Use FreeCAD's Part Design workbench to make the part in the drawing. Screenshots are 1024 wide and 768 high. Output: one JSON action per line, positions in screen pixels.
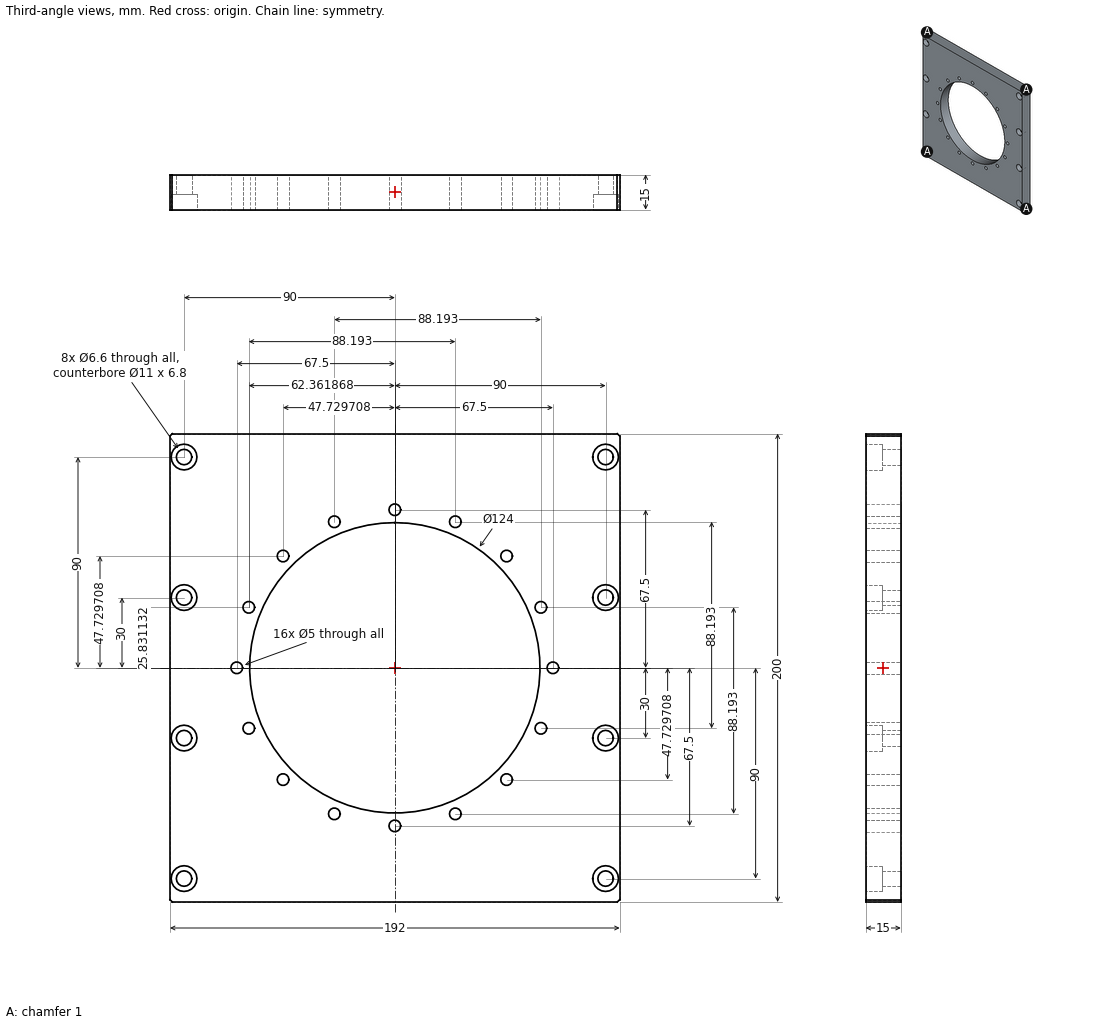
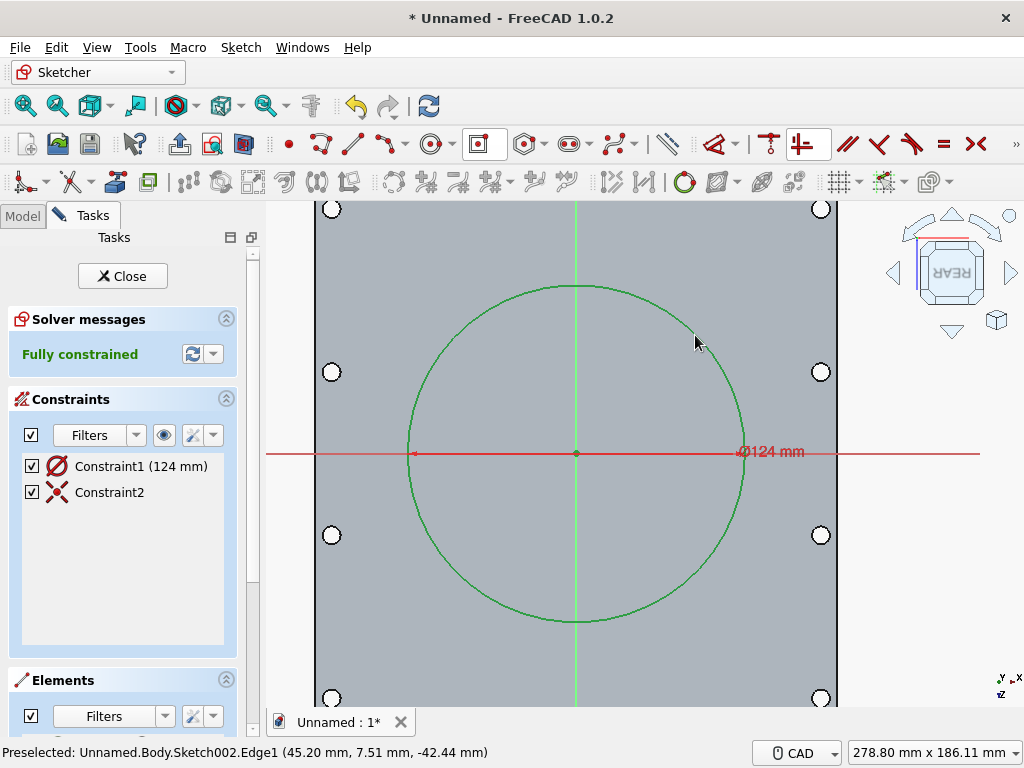
{"action": "left_click", "coordinate": [123, 276]}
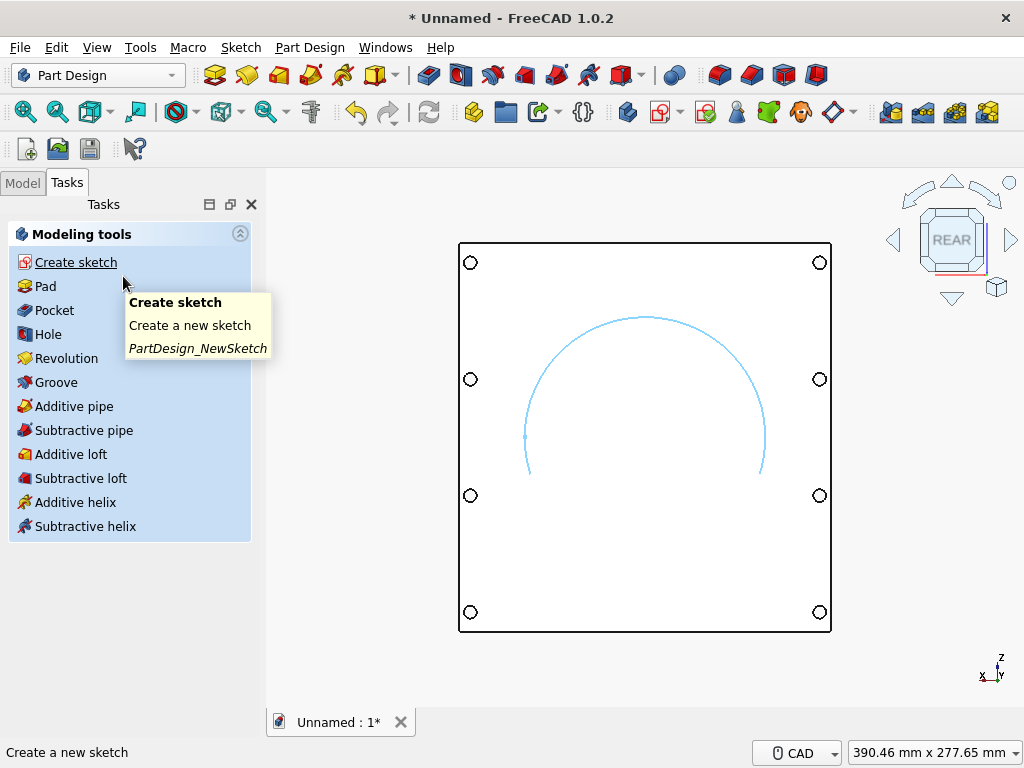
{"action": "left_click", "coordinate": [430, 76]}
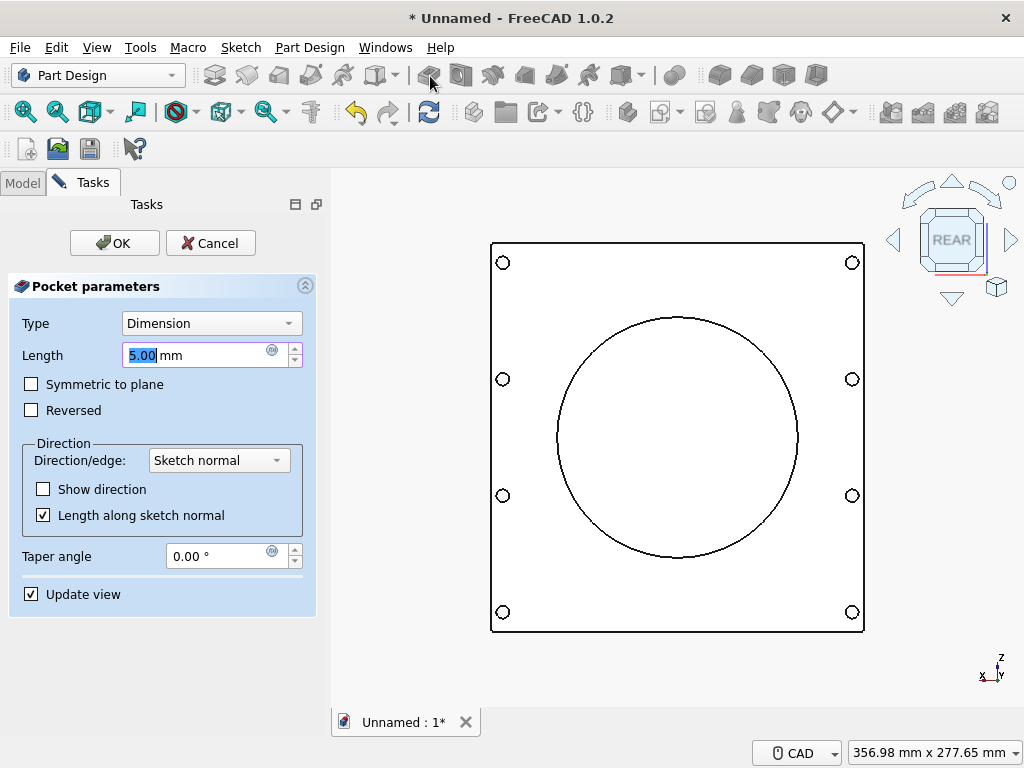
{"action": "type", "text": "15"}
{"action": "key", "text": "Tab"}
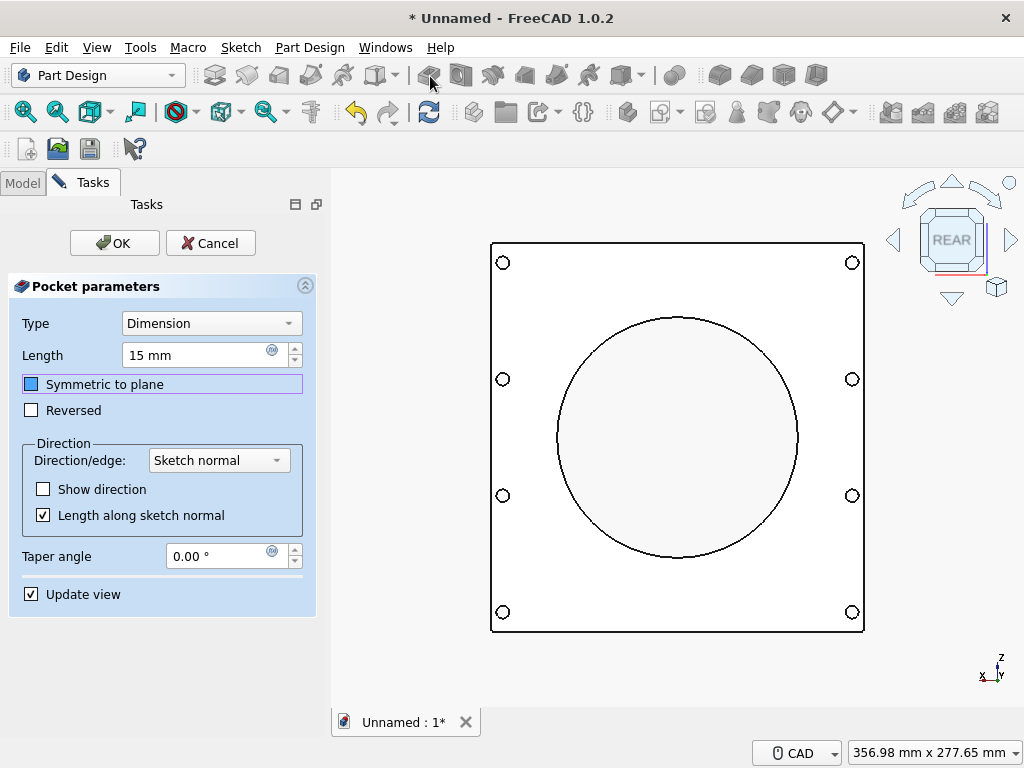
{"action": "left_click", "coordinate": [115, 243]}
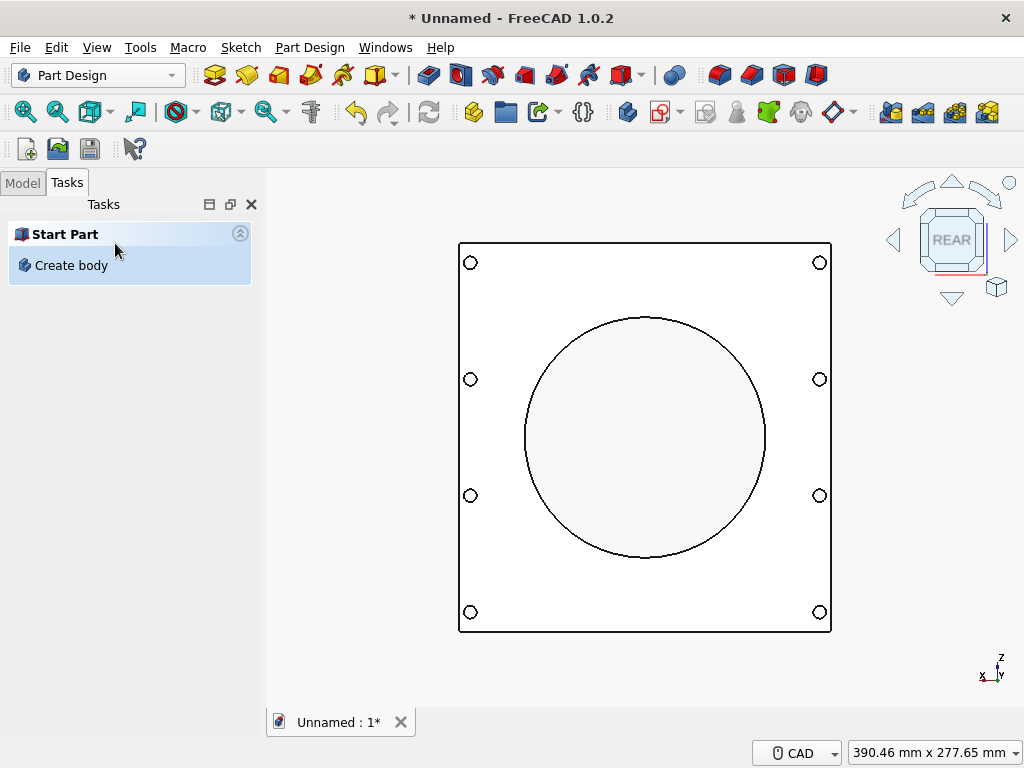
{"action": "key", "text": "0"}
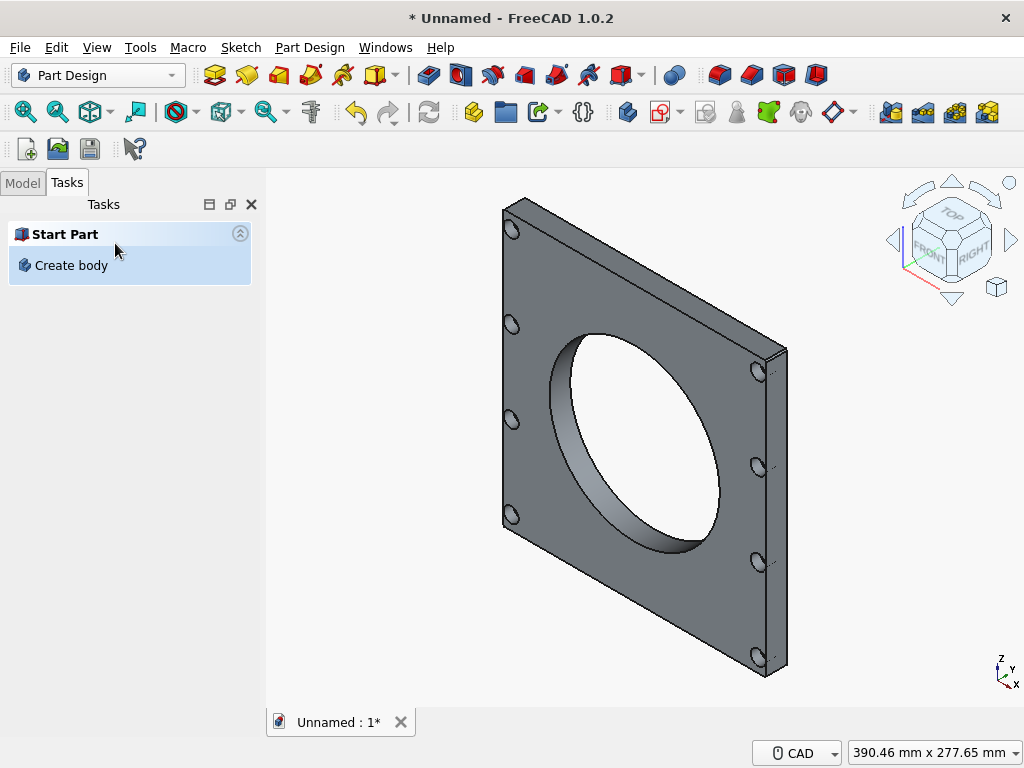
{"action": "left_click", "coordinate": [710, 395]}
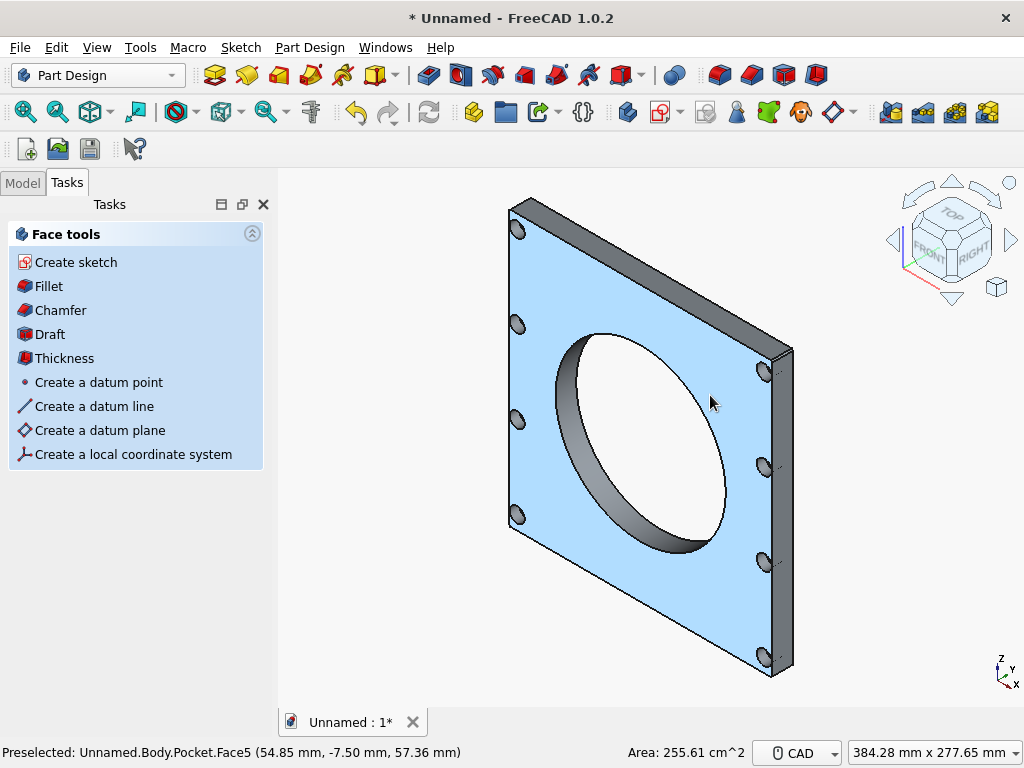
{"action": "left_click", "coordinate": [660, 112]}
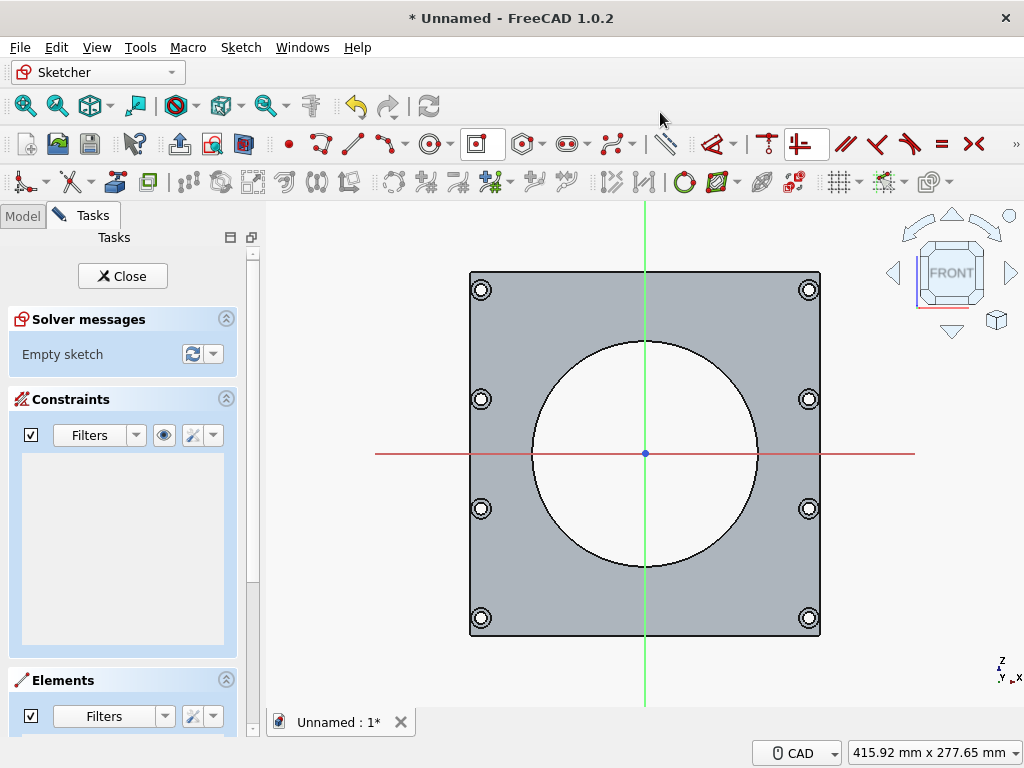
{"action": "left_click", "coordinate": [430, 144]}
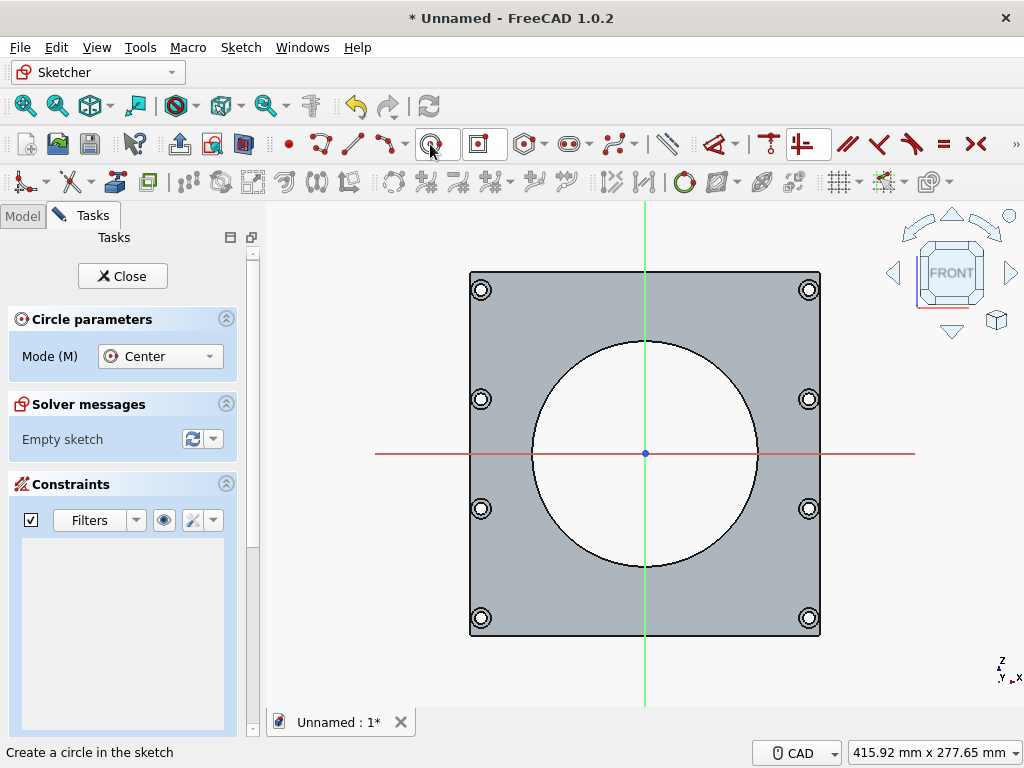
{"action": "scroll", "coordinate": [522, 454], "scroll_direction": "up", "scroll_amount": 9}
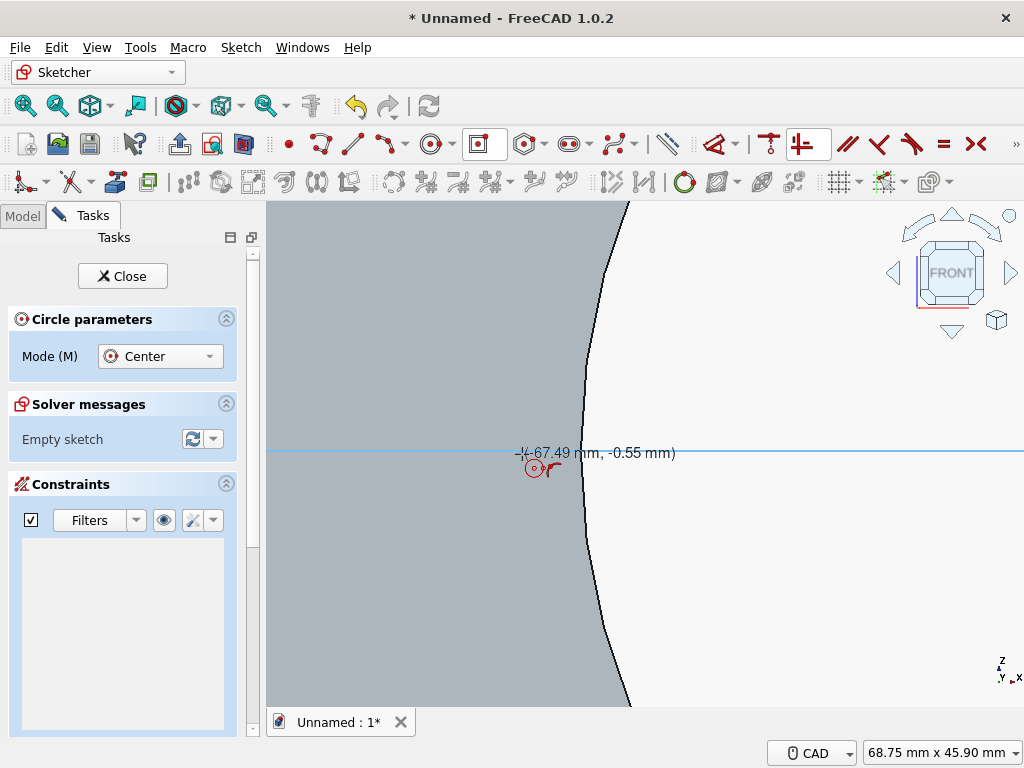
{"action": "scroll", "coordinate": [402, 455], "scroll_direction": "down", "scroll_amount": 8}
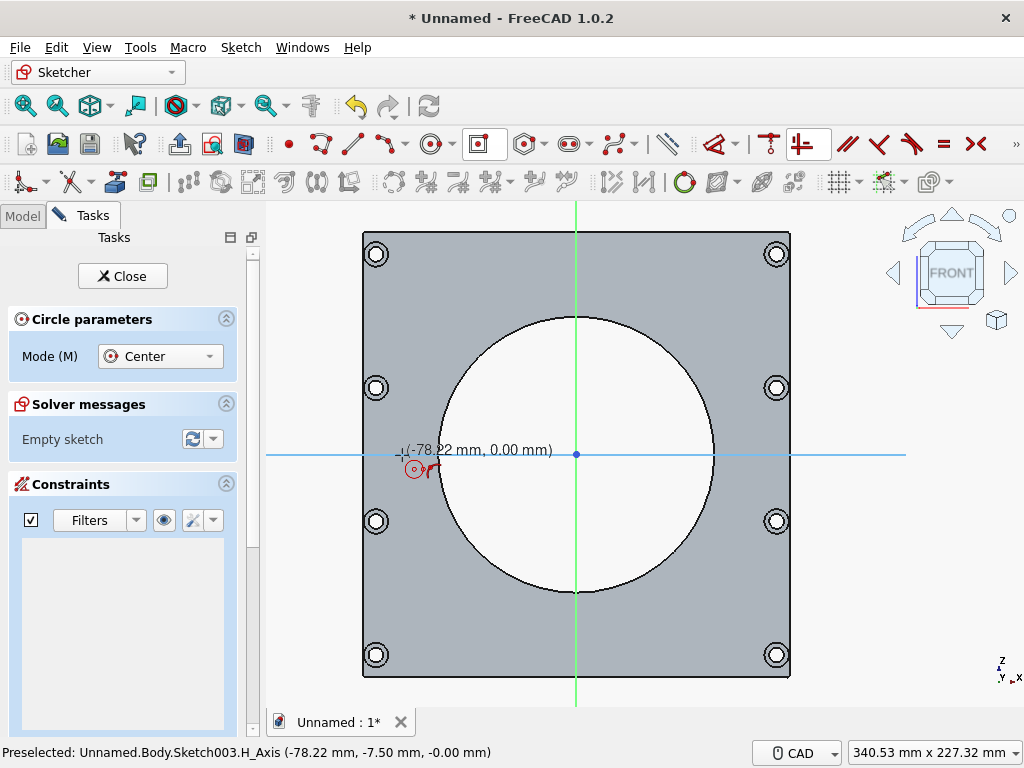
{"action": "left_click", "coordinate": [426, 455]}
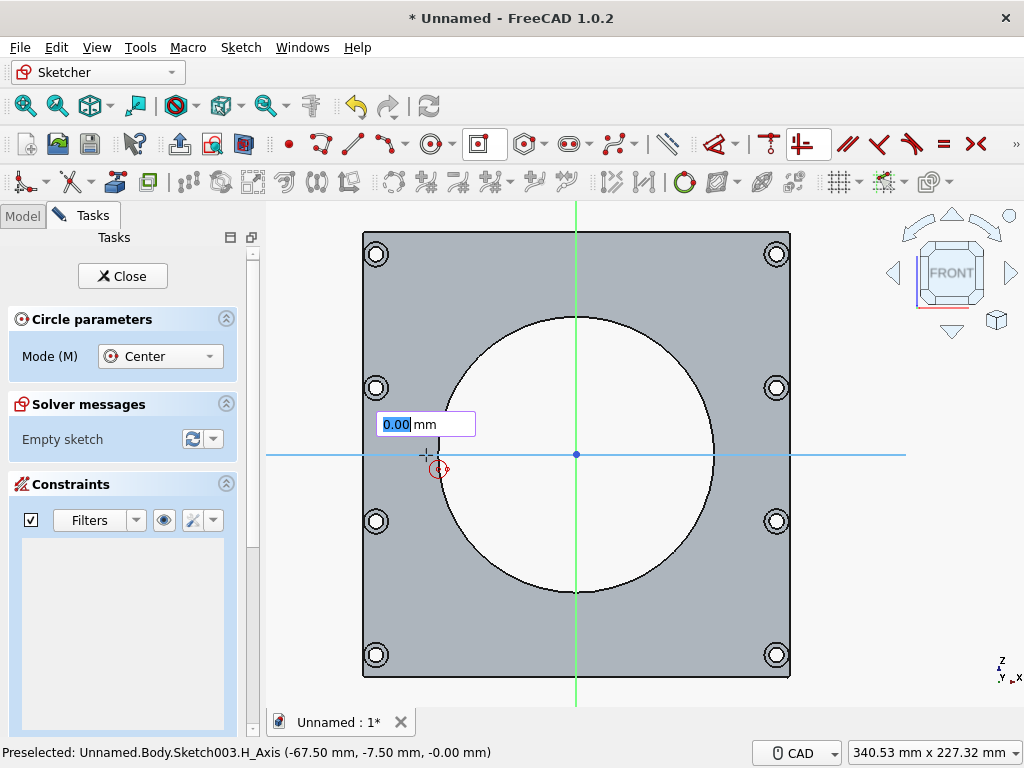
{"action": "scroll", "coordinate": [424, 460], "scroll_direction": "up", "scroll_amount": 6}
{"action": "mouse_move", "coordinate": [424, 459]}